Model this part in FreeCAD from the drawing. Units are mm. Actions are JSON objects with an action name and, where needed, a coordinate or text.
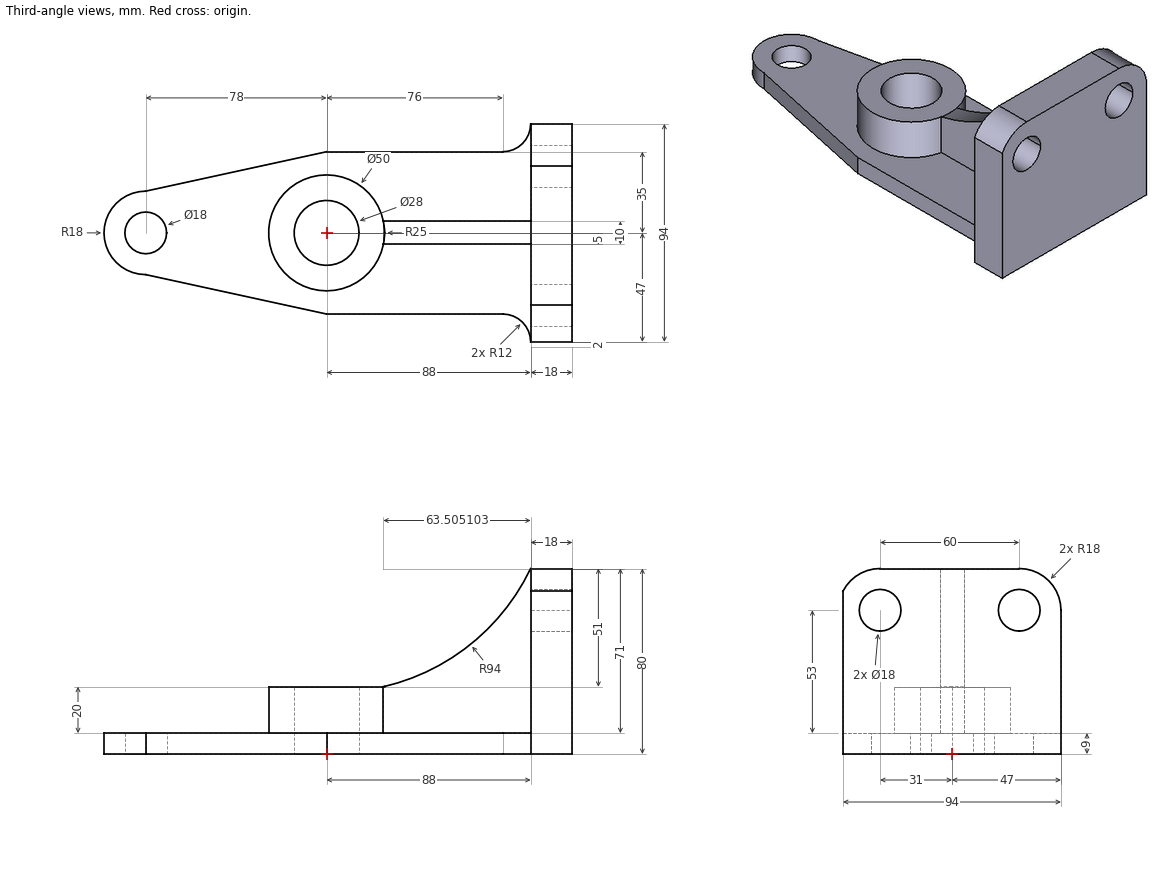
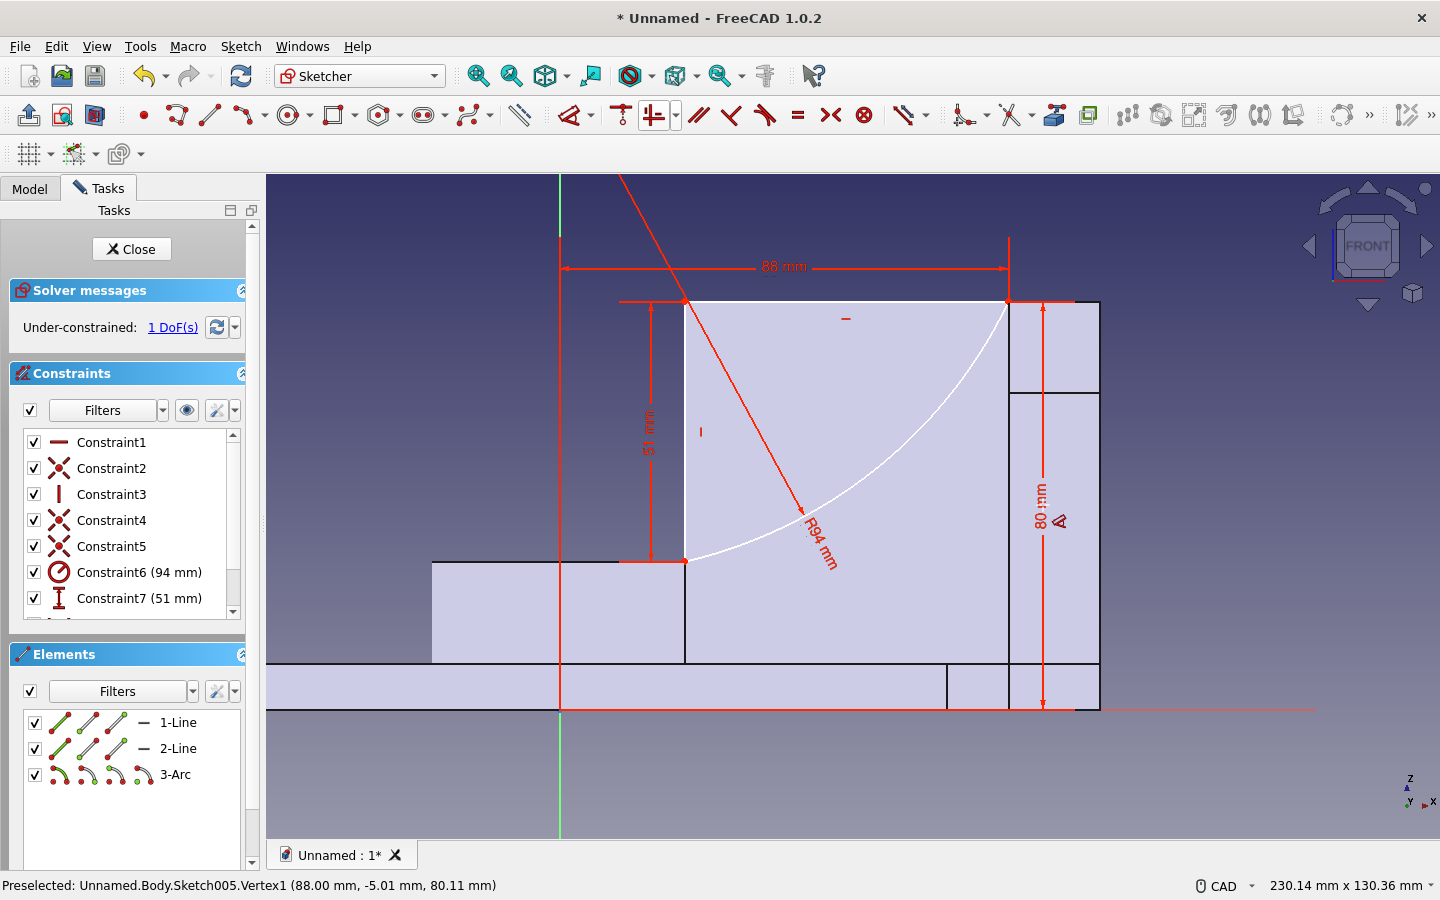
{"action": "left_click", "coordinate": [911, 302]}
{"action": "left_click", "coordinate": [921, 268]}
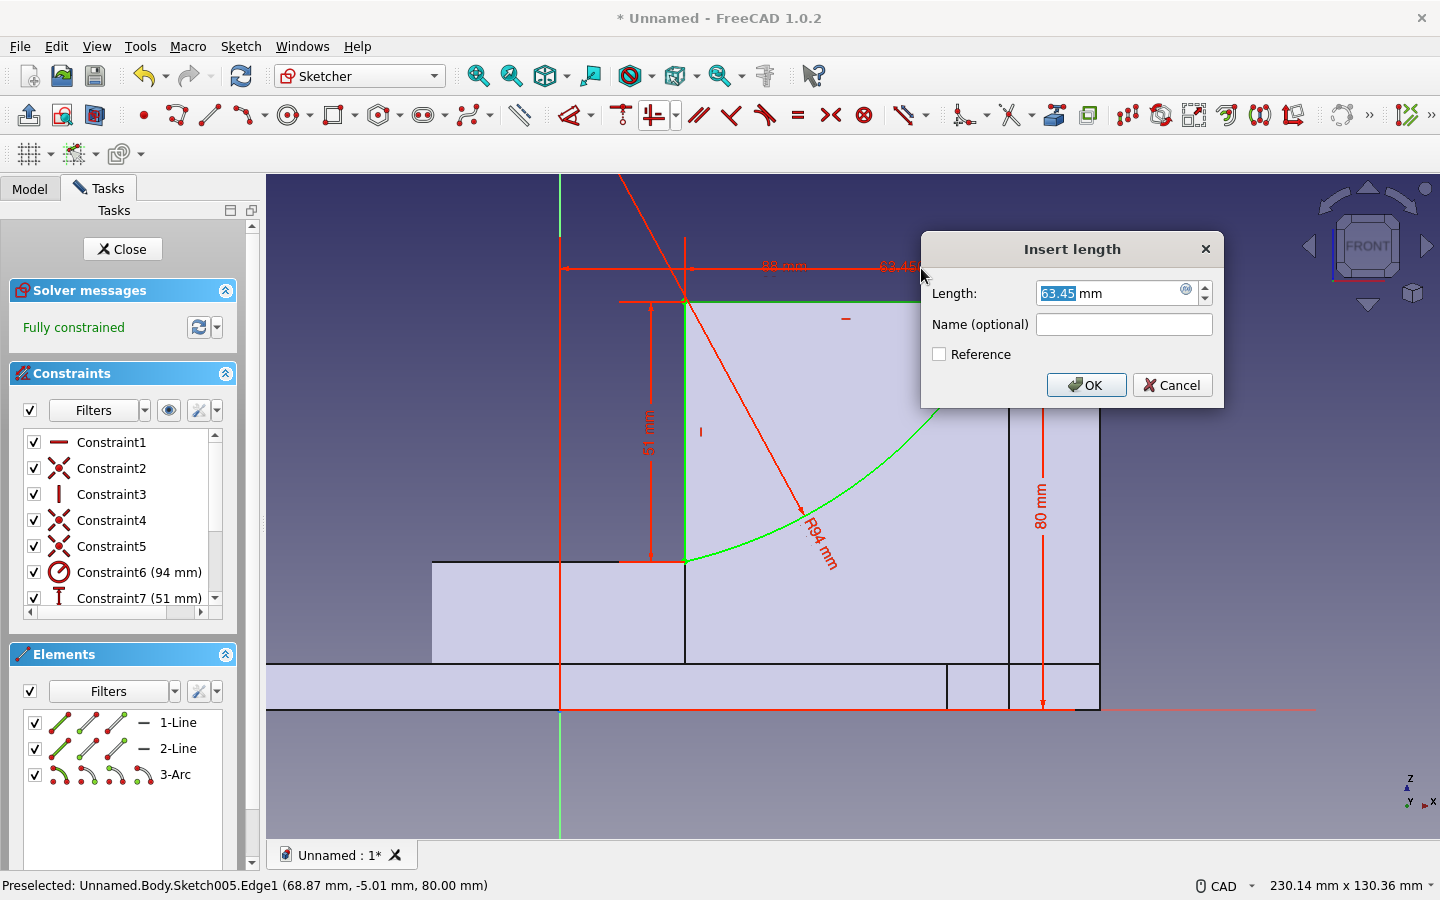
{"action": "type", "text": "63.505103"}
{"action": "key", "text": "Return"}
{"action": "key", "text": "Escape"}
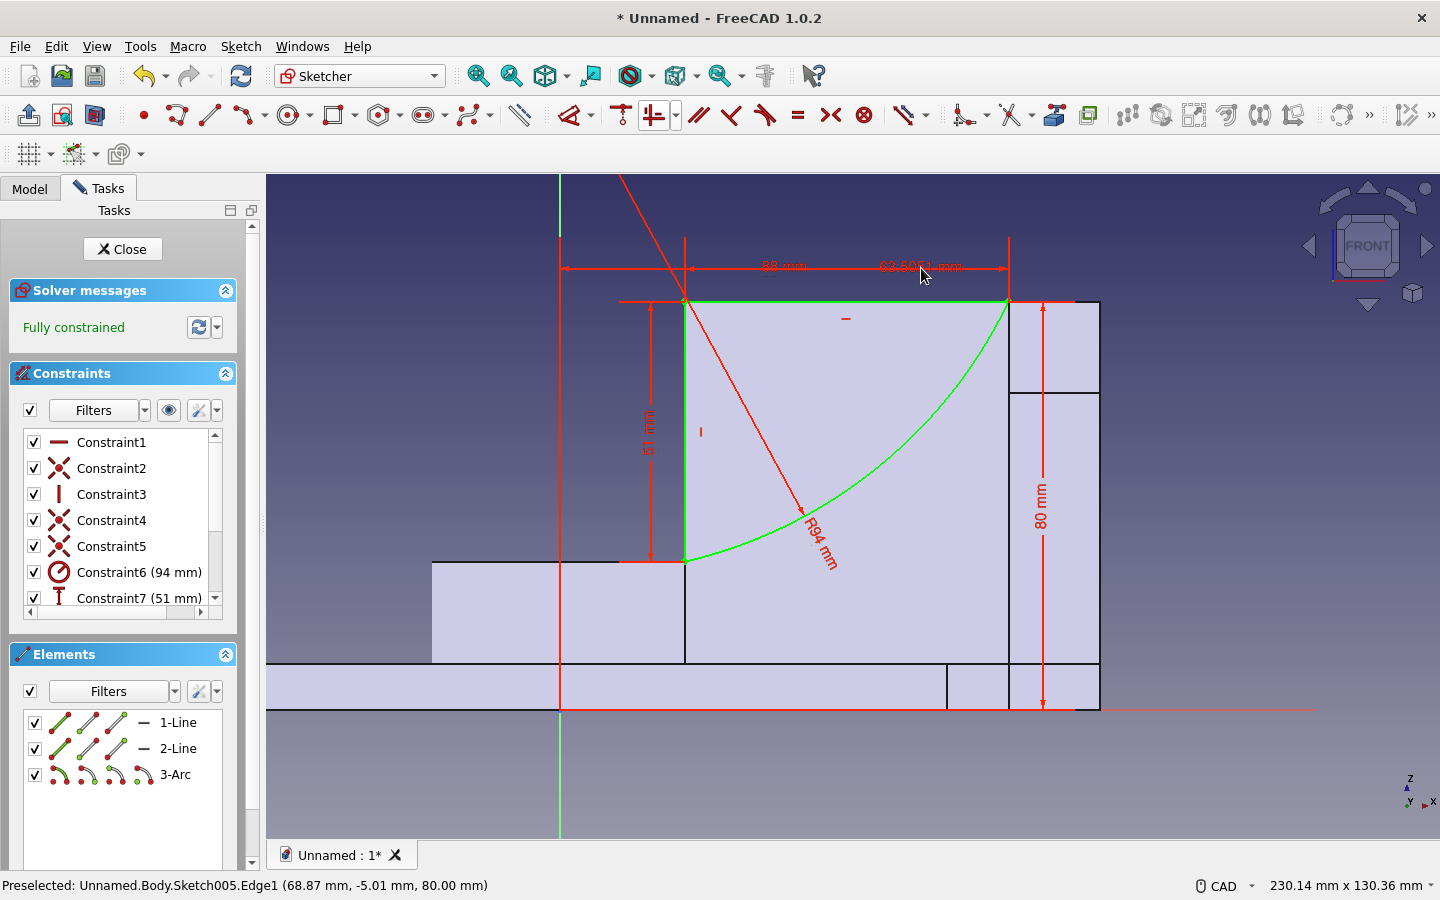
{"action": "left_click", "coordinate": [123, 249]}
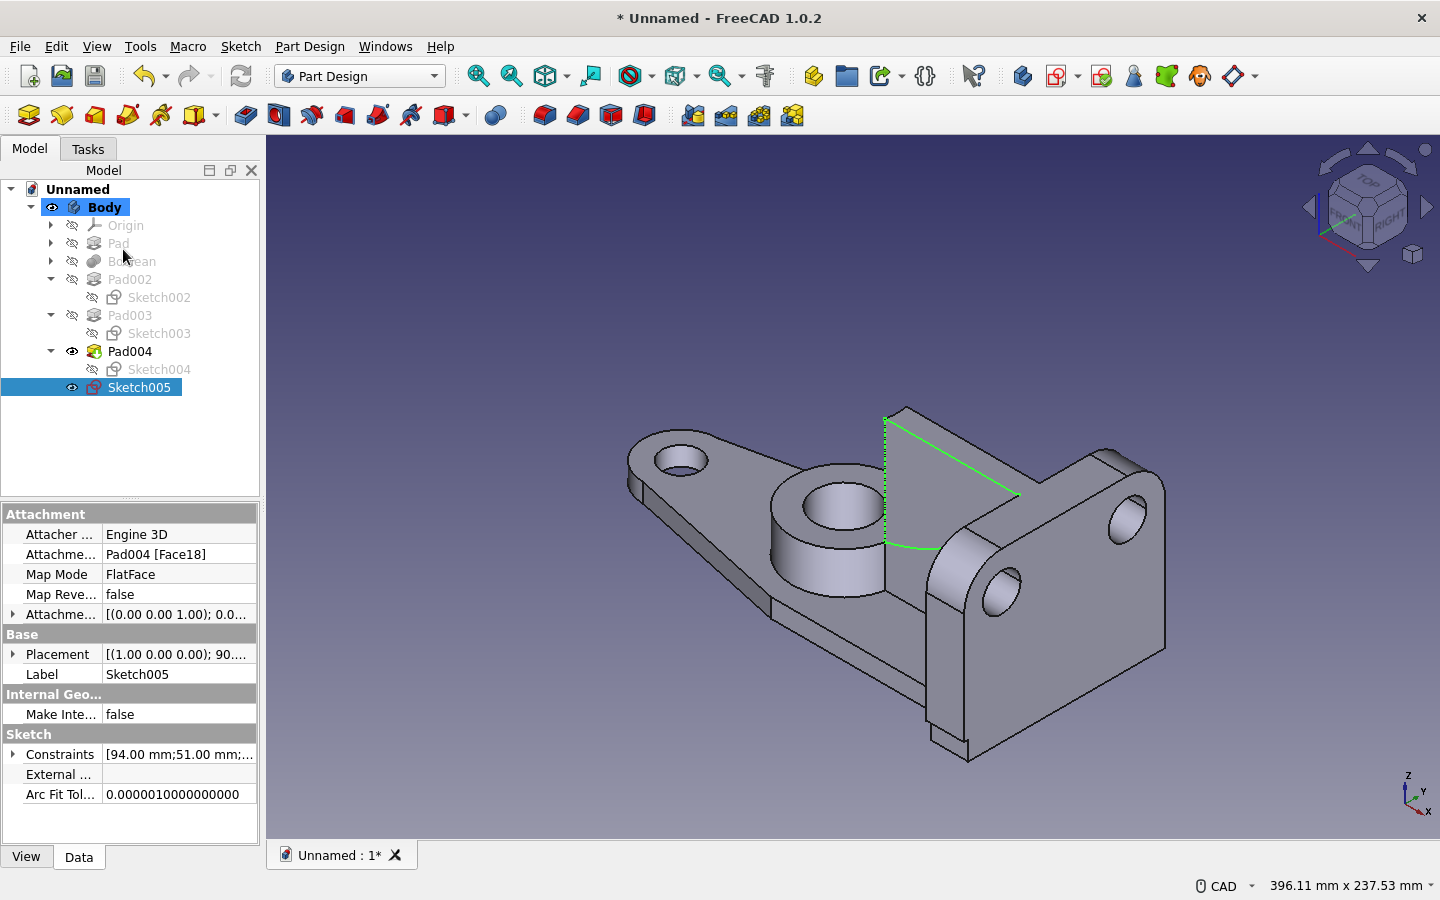
{"action": "left_click", "coordinate": [246, 116]}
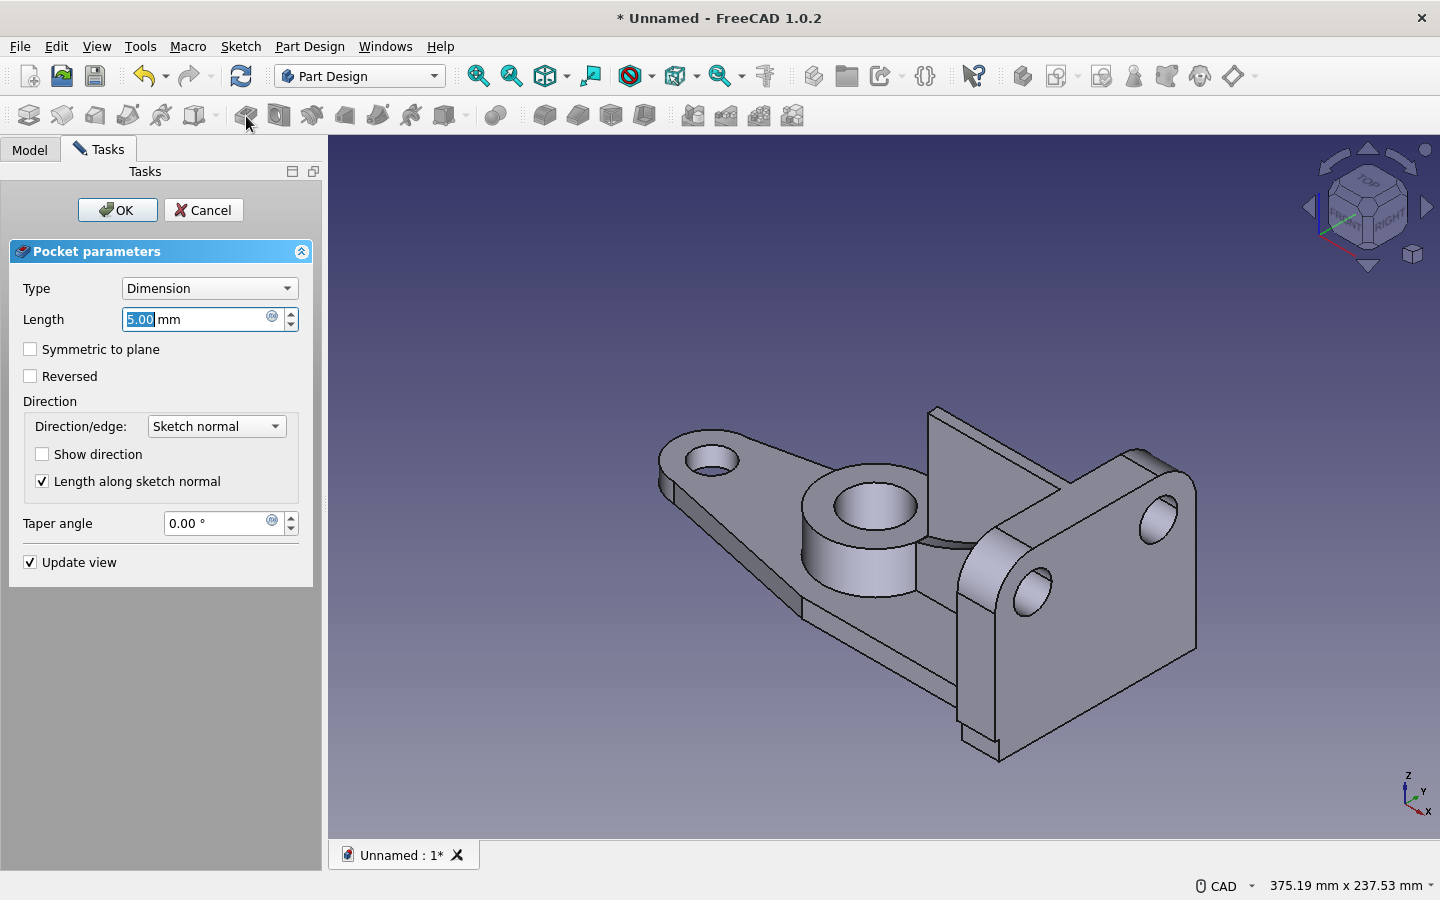
{"action": "left_click", "coordinate": [210, 288]}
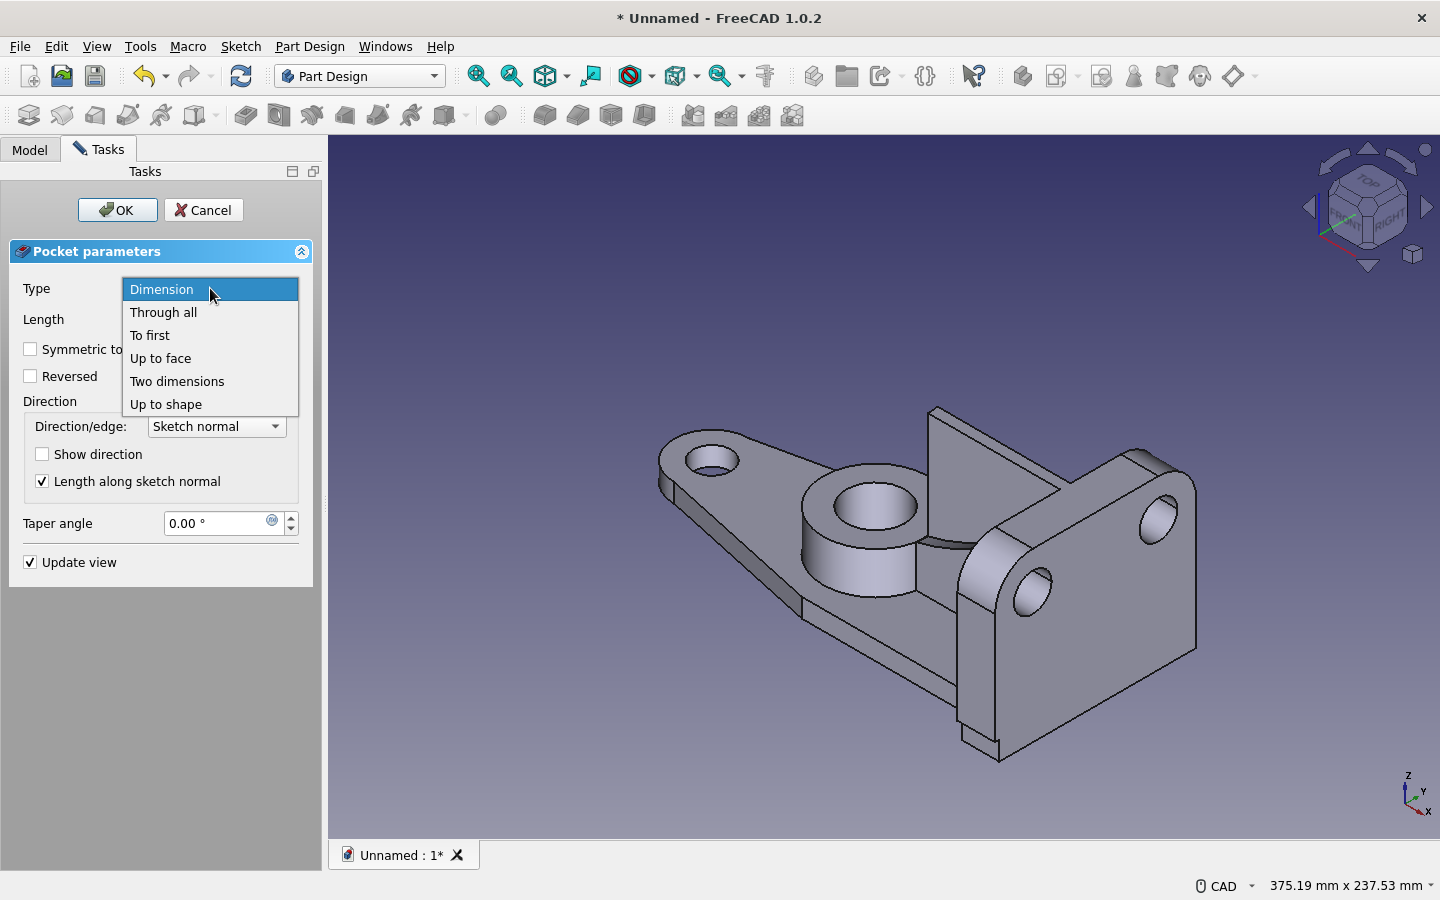
{"action": "left_click", "coordinate": [208, 312]}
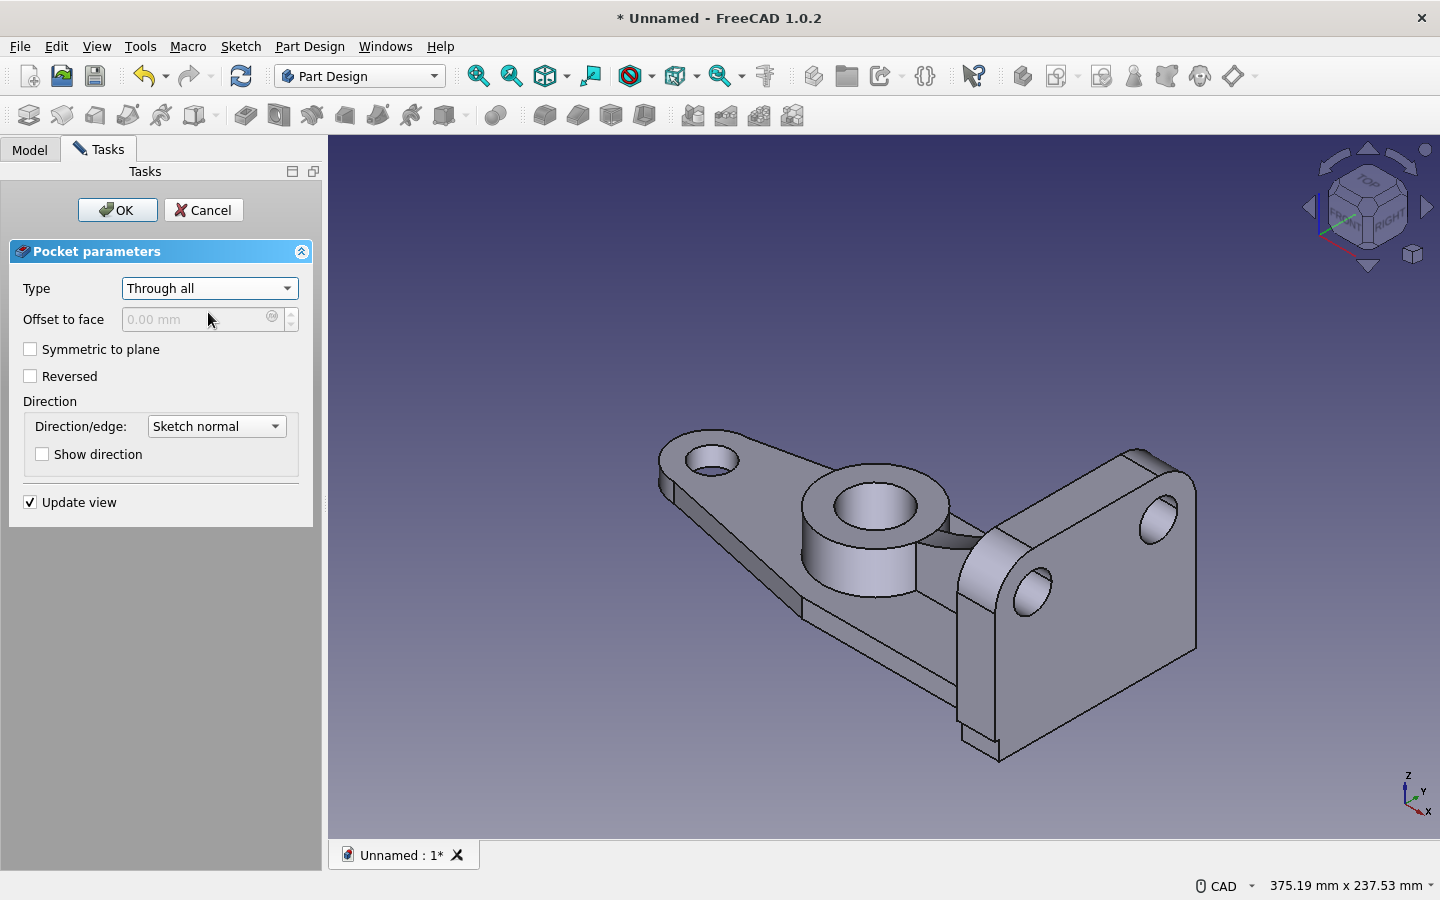
{"action": "left_click", "coordinate": [118, 210]}